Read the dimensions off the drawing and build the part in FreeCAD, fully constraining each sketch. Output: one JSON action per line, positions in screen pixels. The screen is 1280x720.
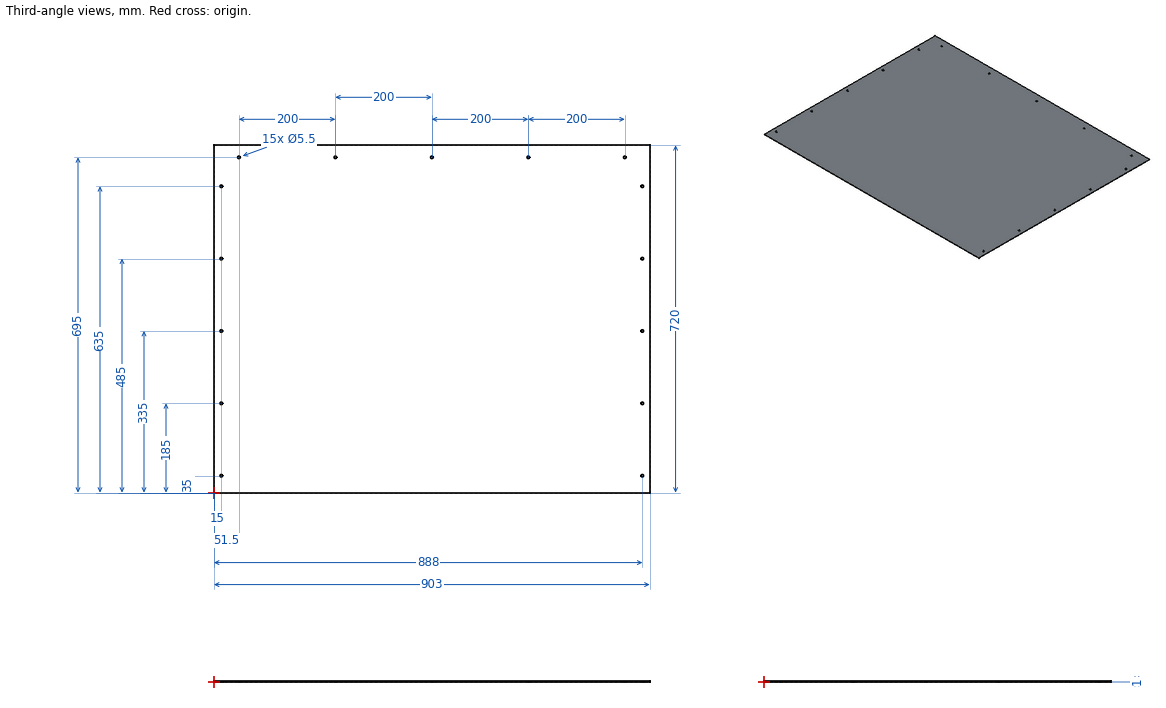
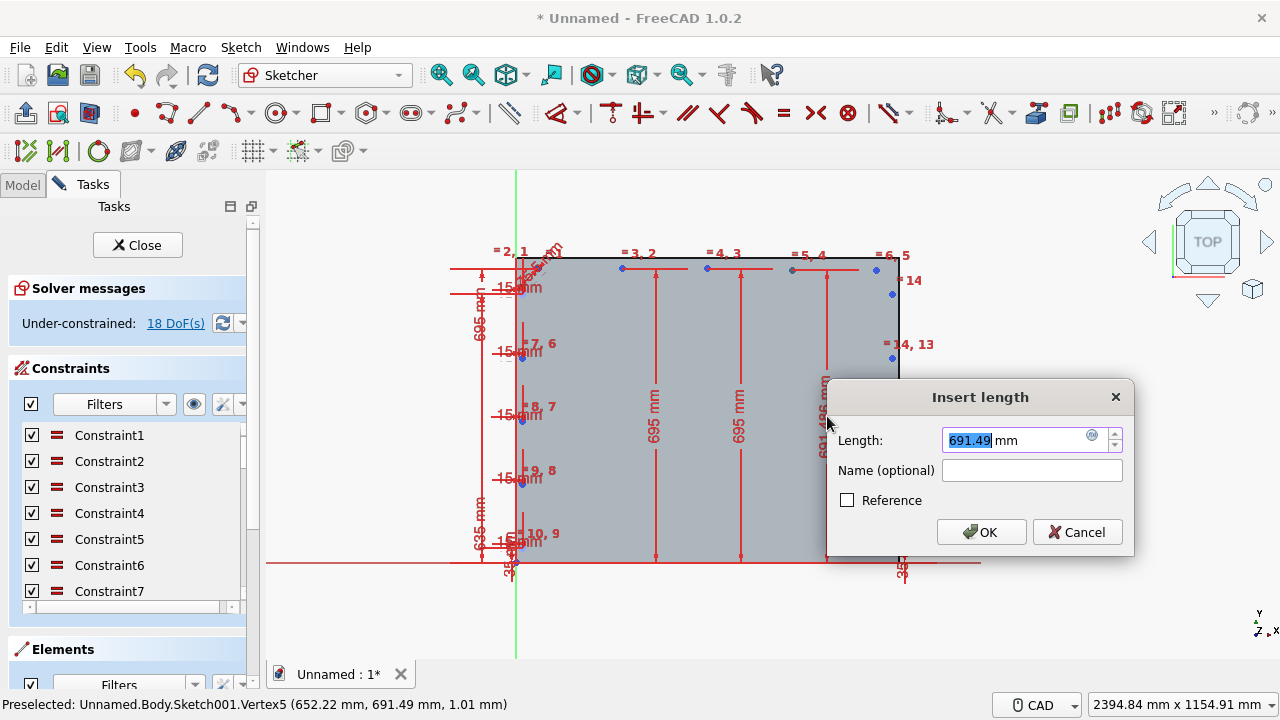
{"action": "type", "text": "695"}
{"action": "key", "text": "Return"}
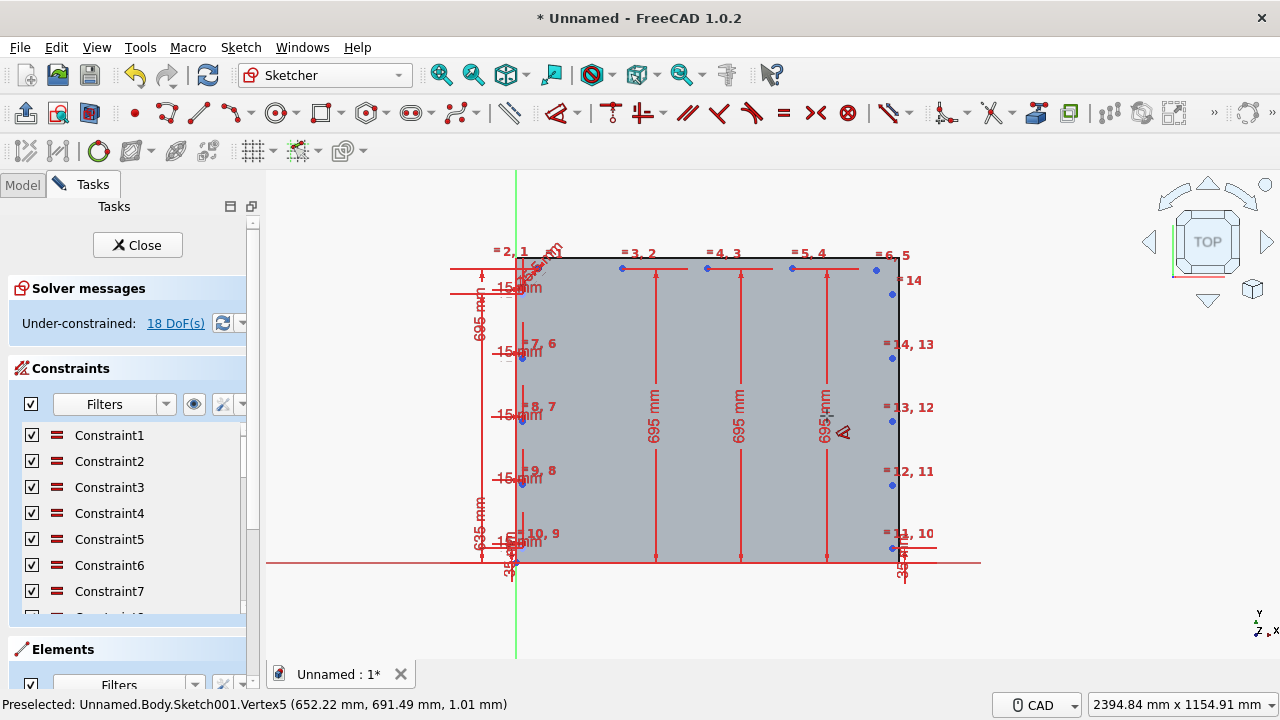
{"action": "left_click", "coordinate": [877, 270]}
{"action": "left_click", "coordinate": [911, 416]}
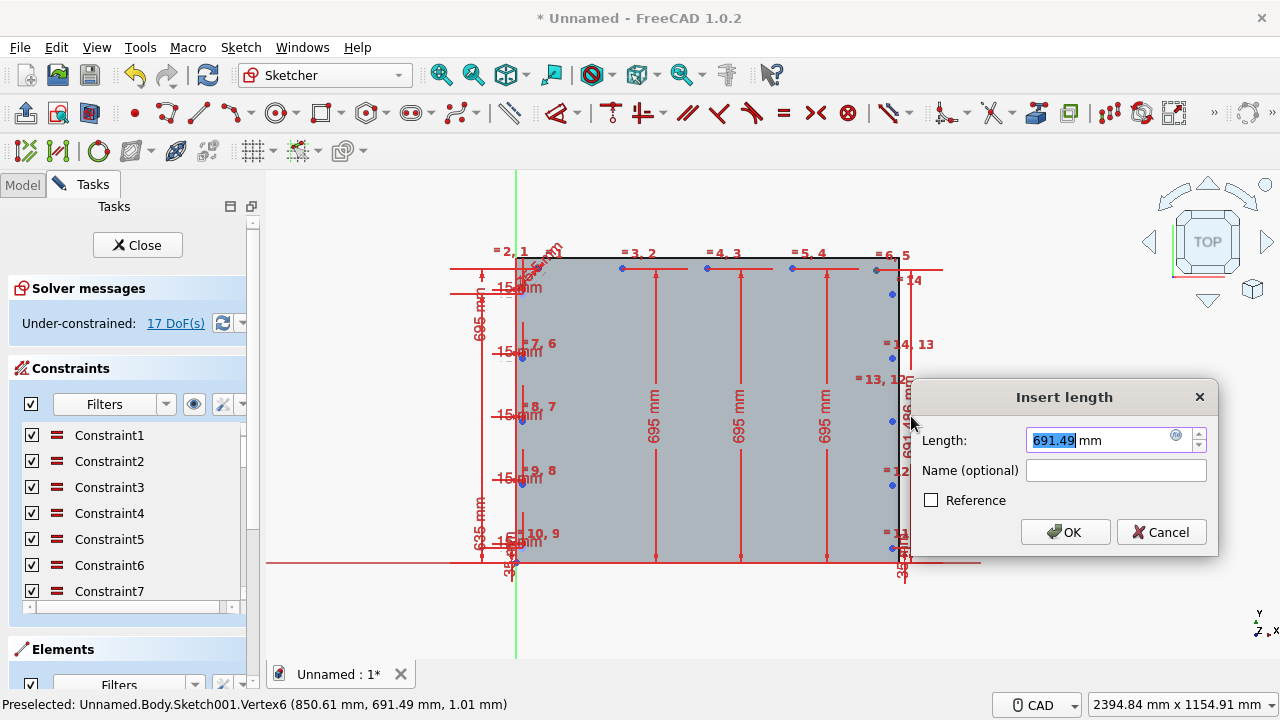
{"action": "type", "text": "695"}
{"action": "key", "text": "Return"}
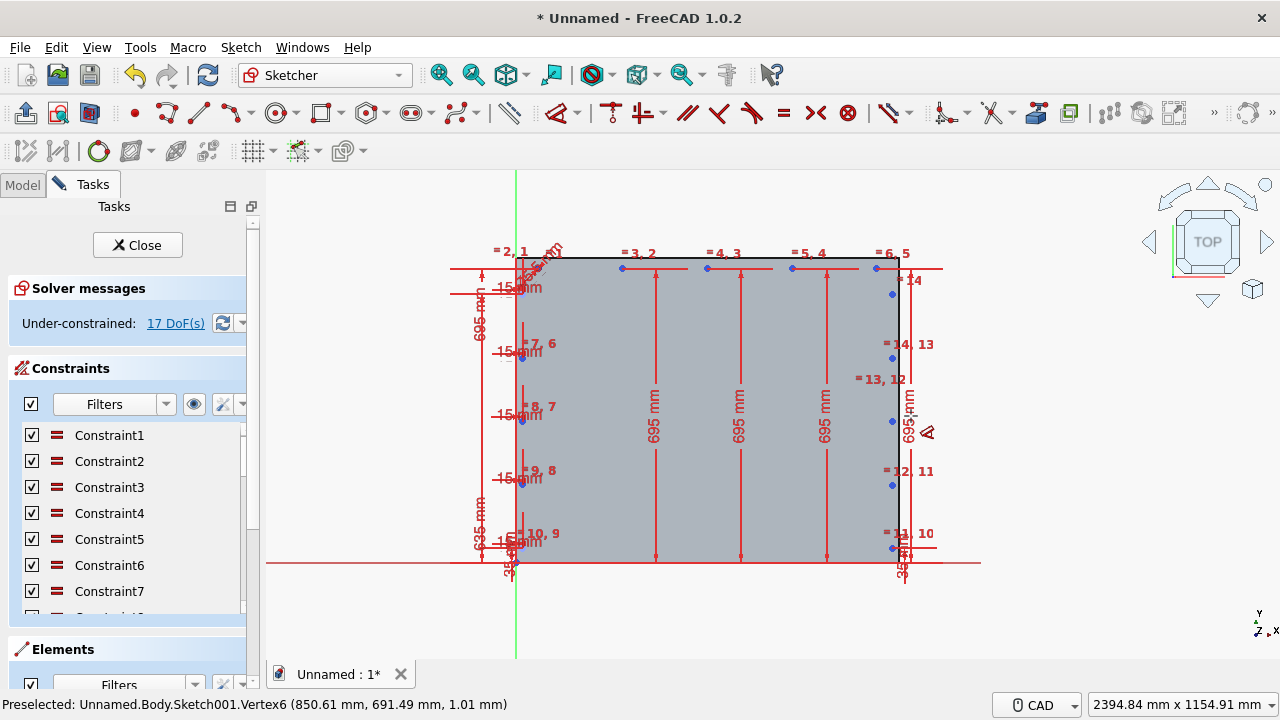
{"action": "left_click", "coordinate": [523, 358]}
{"action": "left_click", "coordinate": [482, 389]}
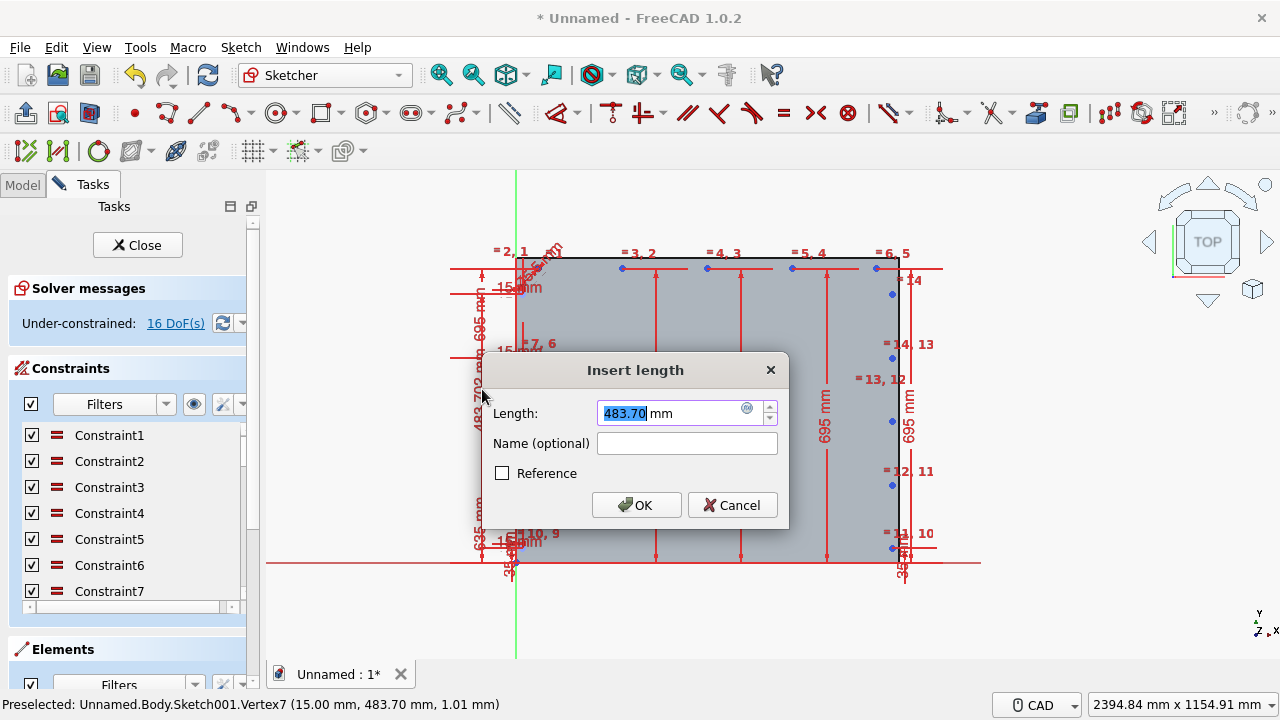
{"action": "type", "text": "485"}
{"action": "key", "text": "Return"}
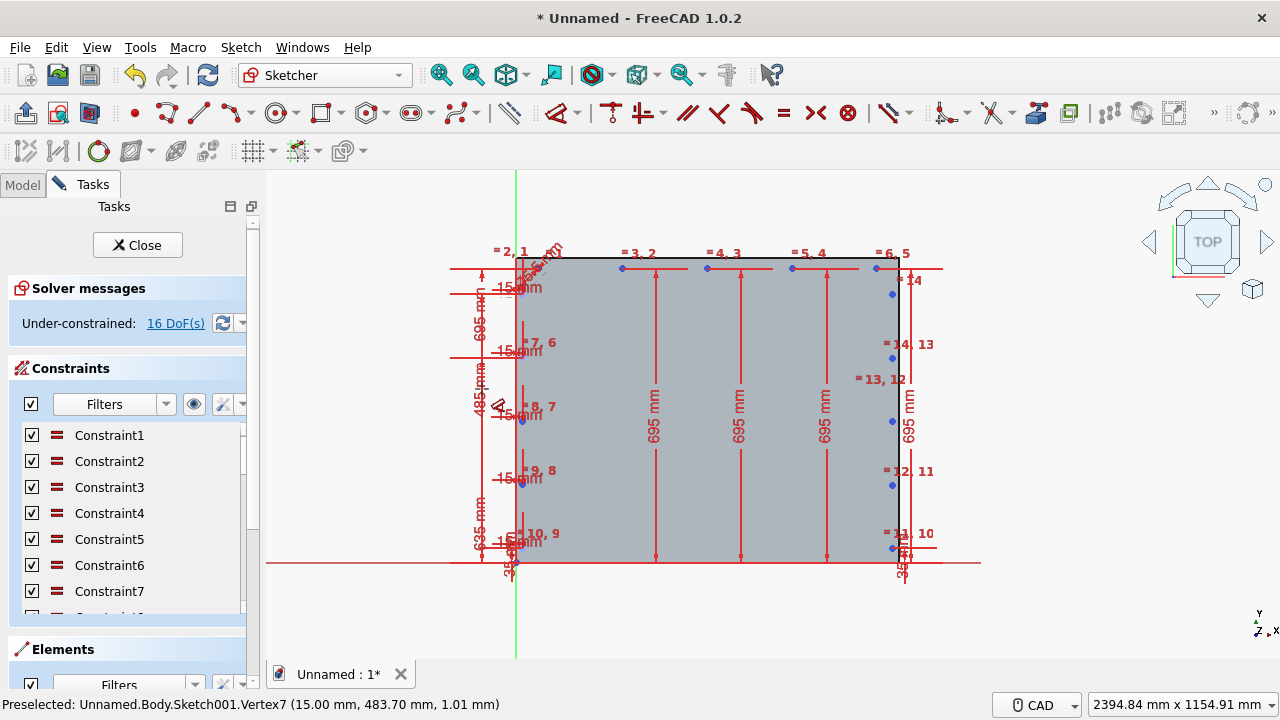
{"action": "left_click", "coordinate": [523, 421]}
{"action": "left_click", "coordinate": [482, 460]}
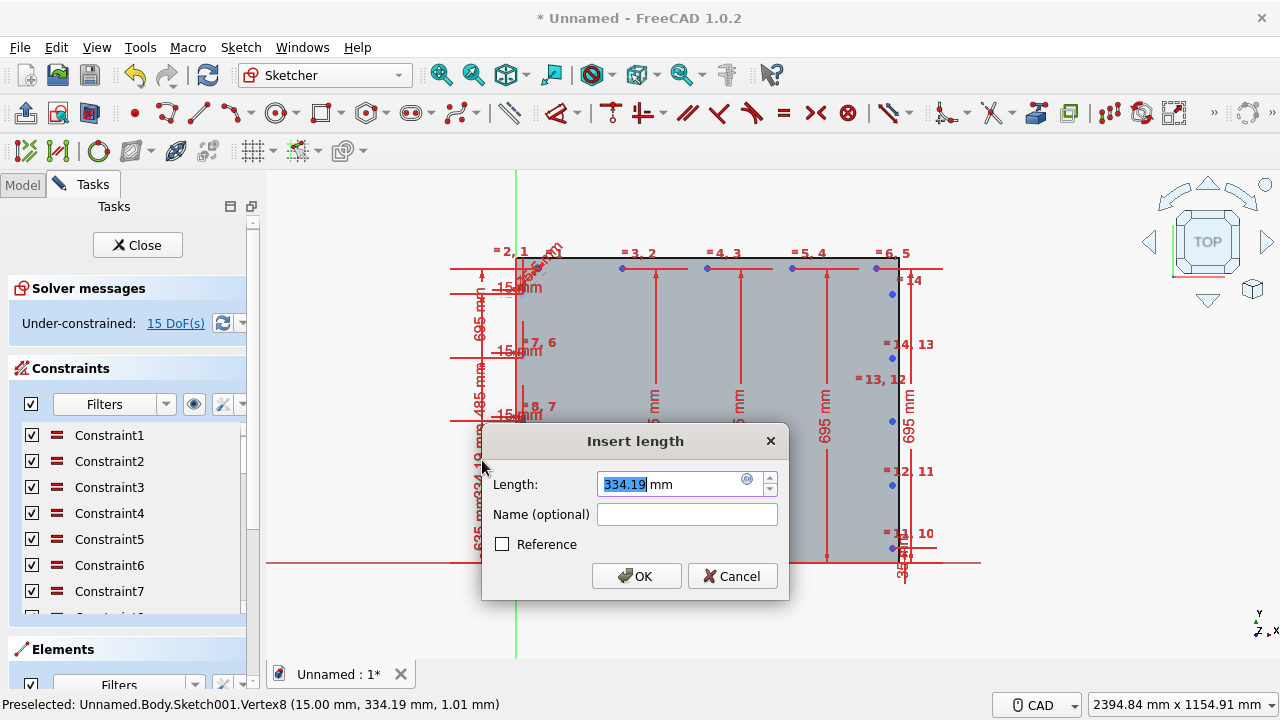
{"action": "type", "text": "335"}
{"action": "key", "text": "Return"}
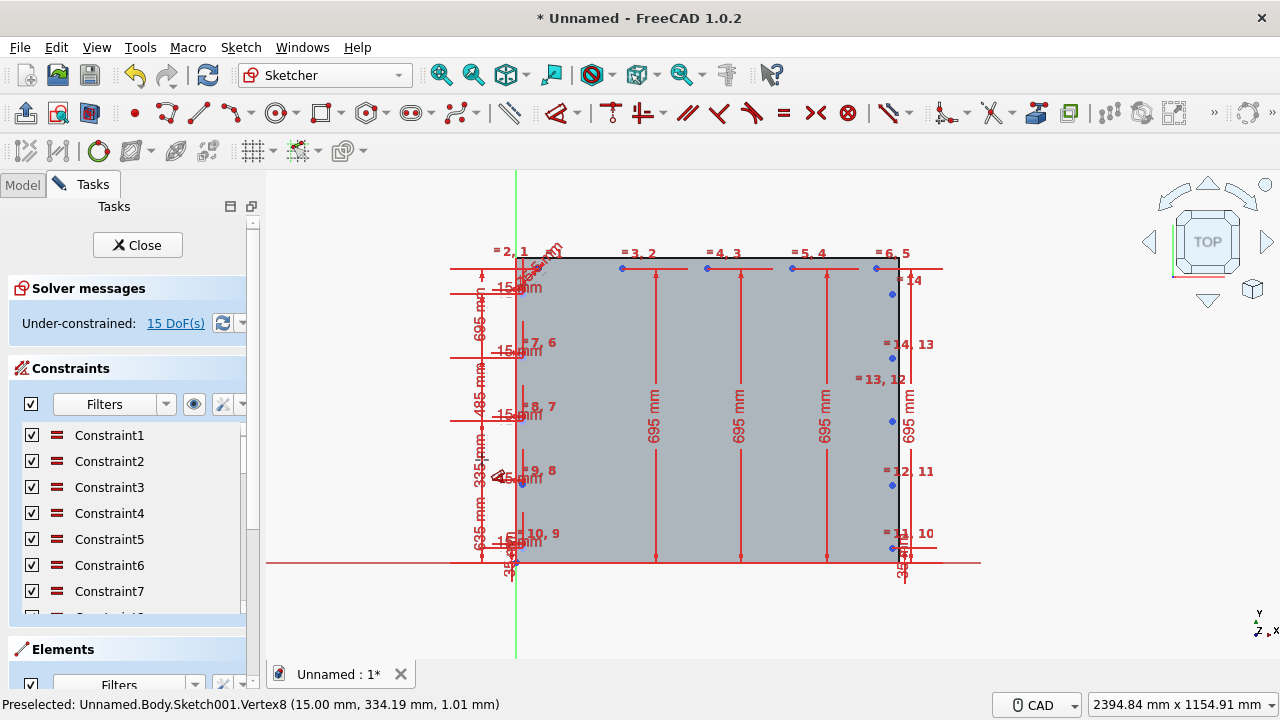
{"action": "left_click", "coordinate": [523, 485]}
{"action": "left_click", "coordinate": [557, 506]}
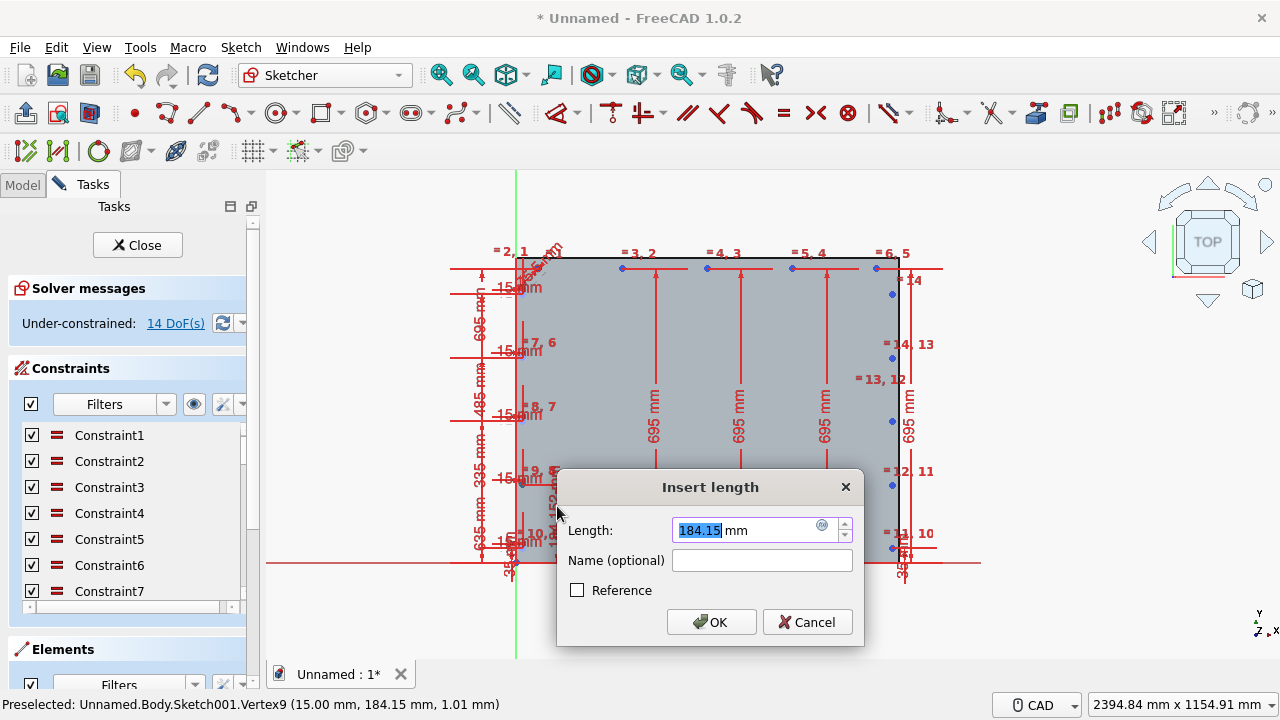
{"action": "type", "text": "185"}
{"action": "key", "text": "Return"}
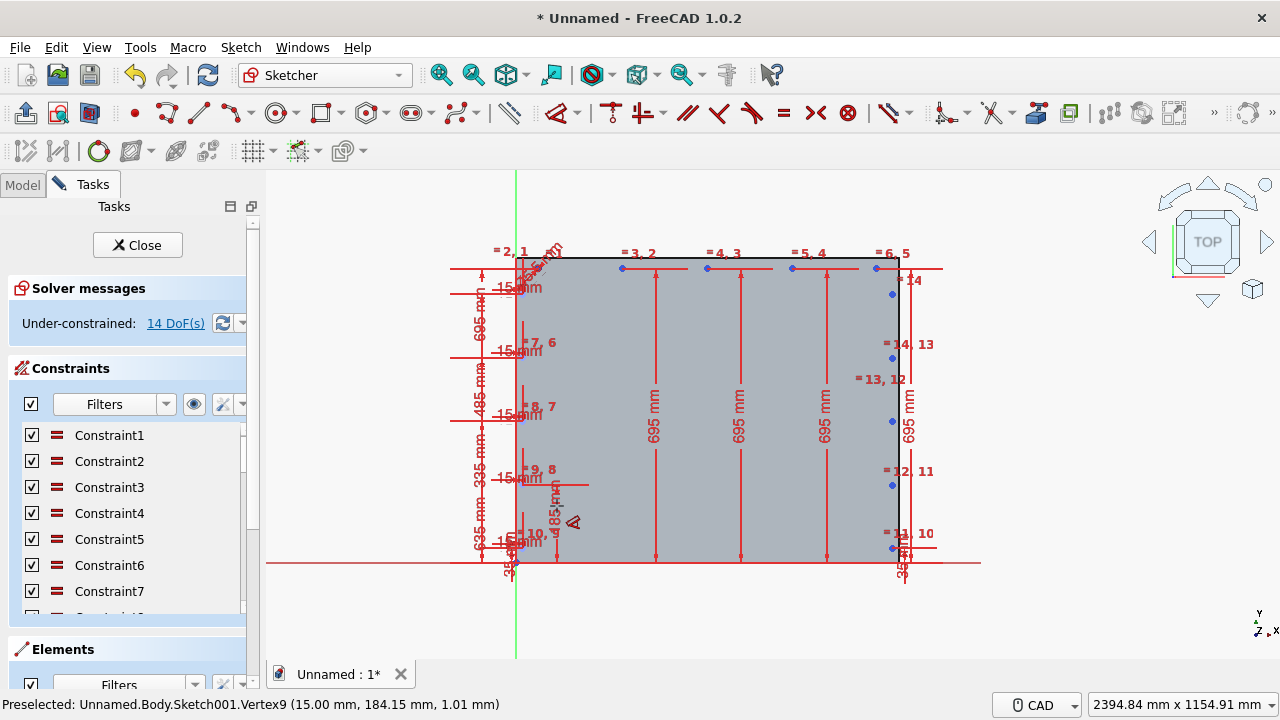
{"action": "left_click", "coordinate": [892, 548]}
{"action": "left_click", "coordinate": [704, 597]}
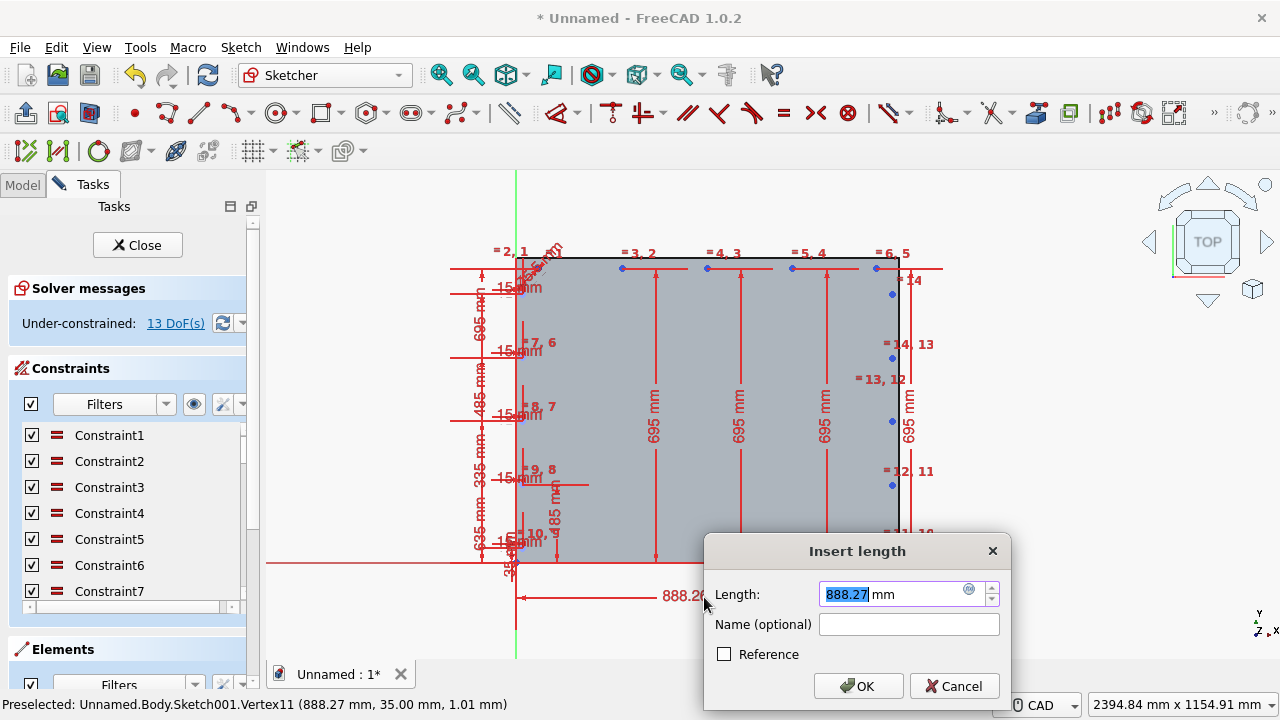
{"action": "type", "text": "888"}
{"action": "key", "text": "Return"}